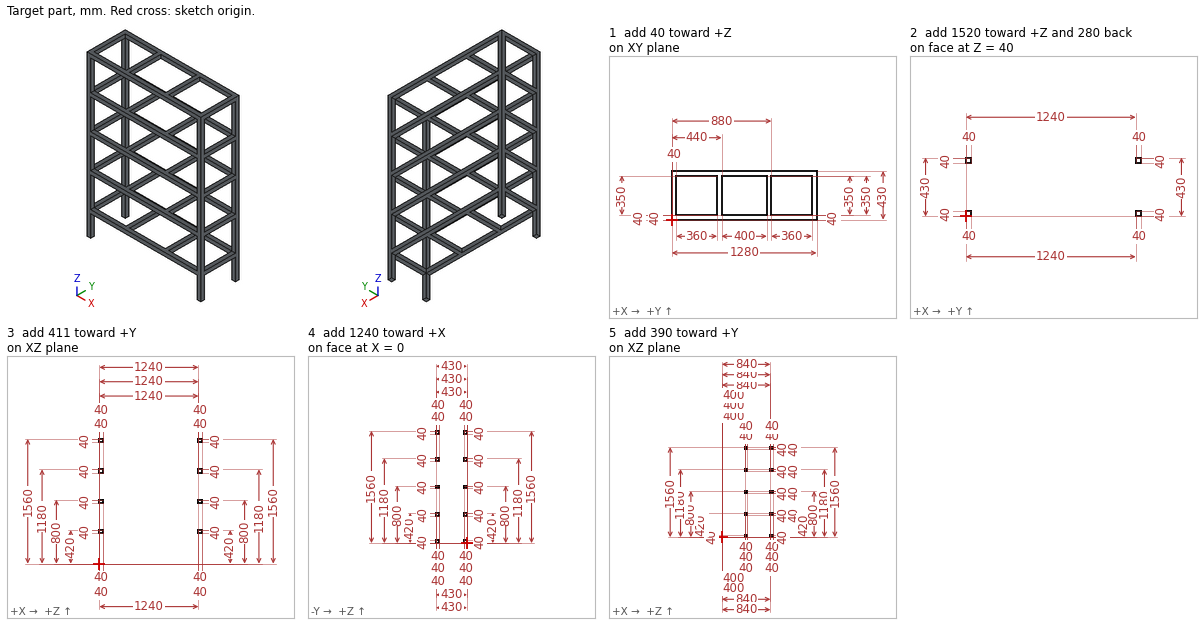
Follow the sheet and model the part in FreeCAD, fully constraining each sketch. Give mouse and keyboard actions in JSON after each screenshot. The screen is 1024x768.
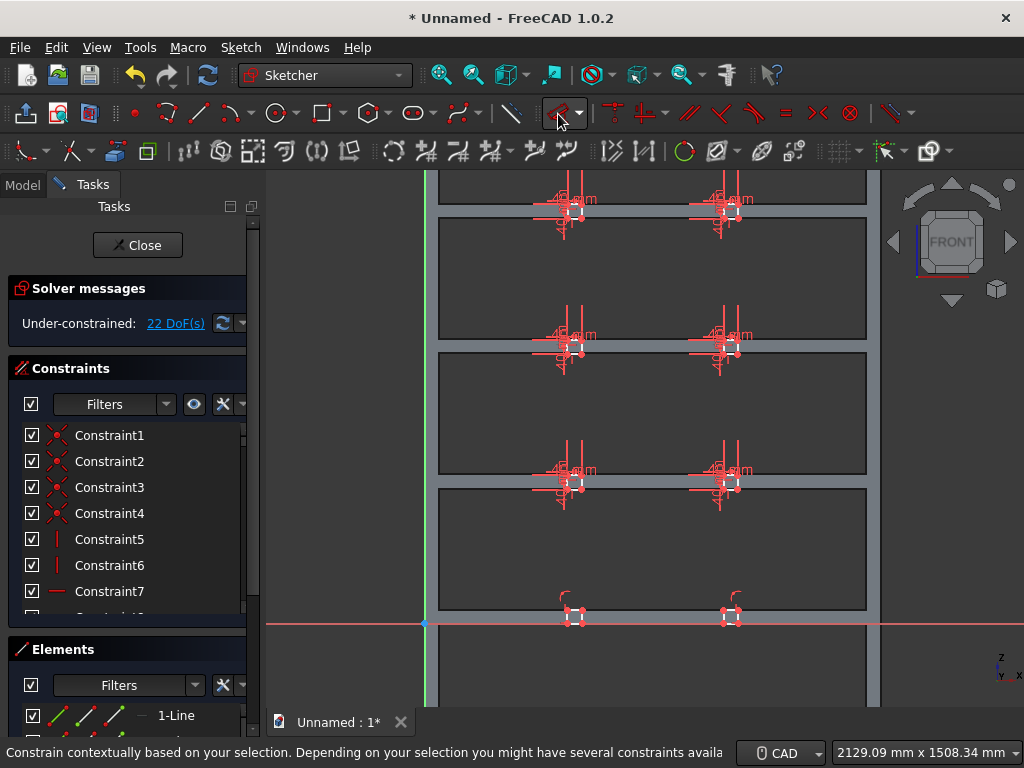
{"action": "scroll", "coordinate": [567, 617], "scroll_direction": "up", "scroll_amount": 6}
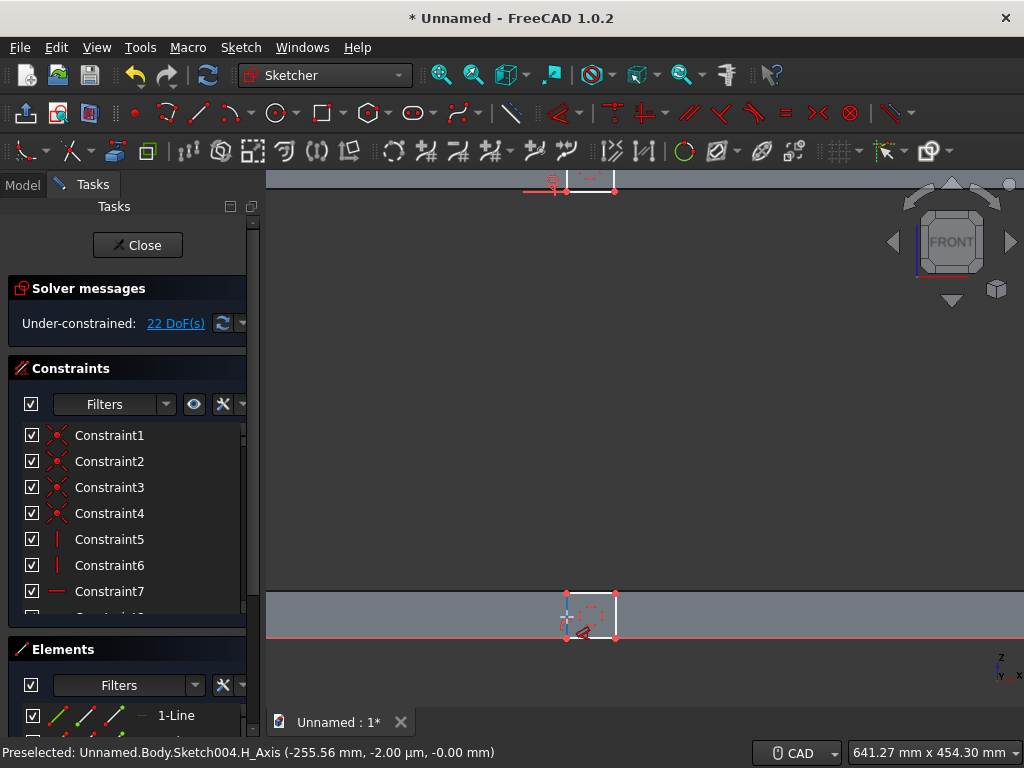
{"action": "left_click", "coordinate": [567, 616]}
{"action": "left_click", "coordinate": [533, 616]}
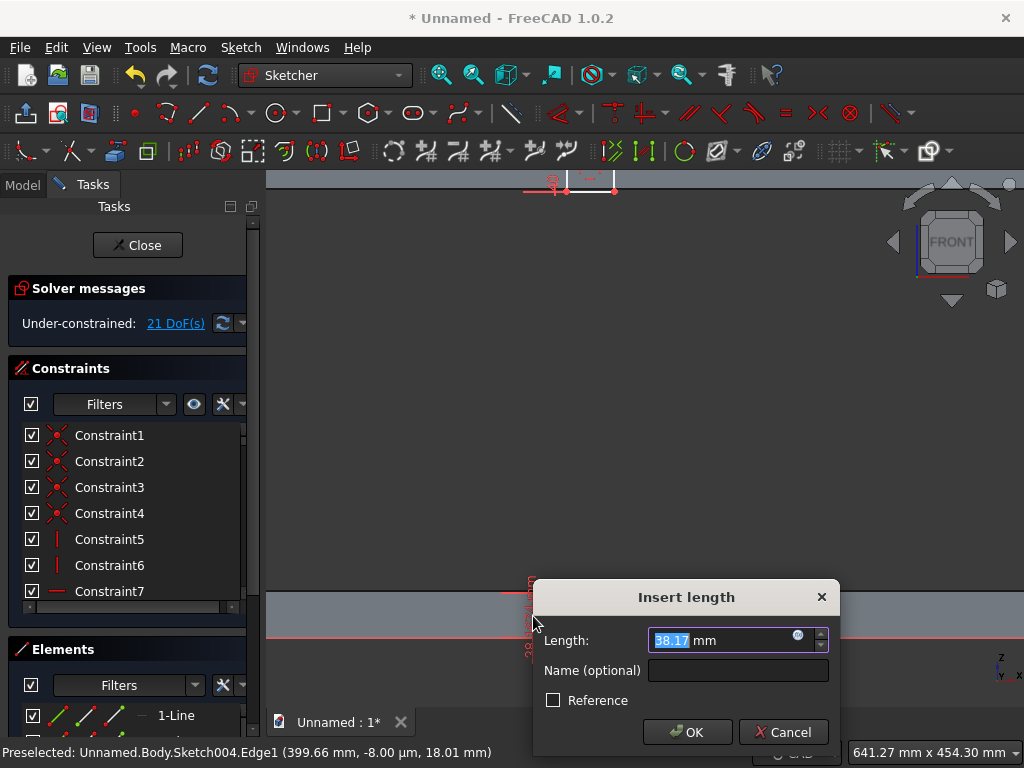
{"action": "type", "text": "40"}
{"action": "key", "text": "Return"}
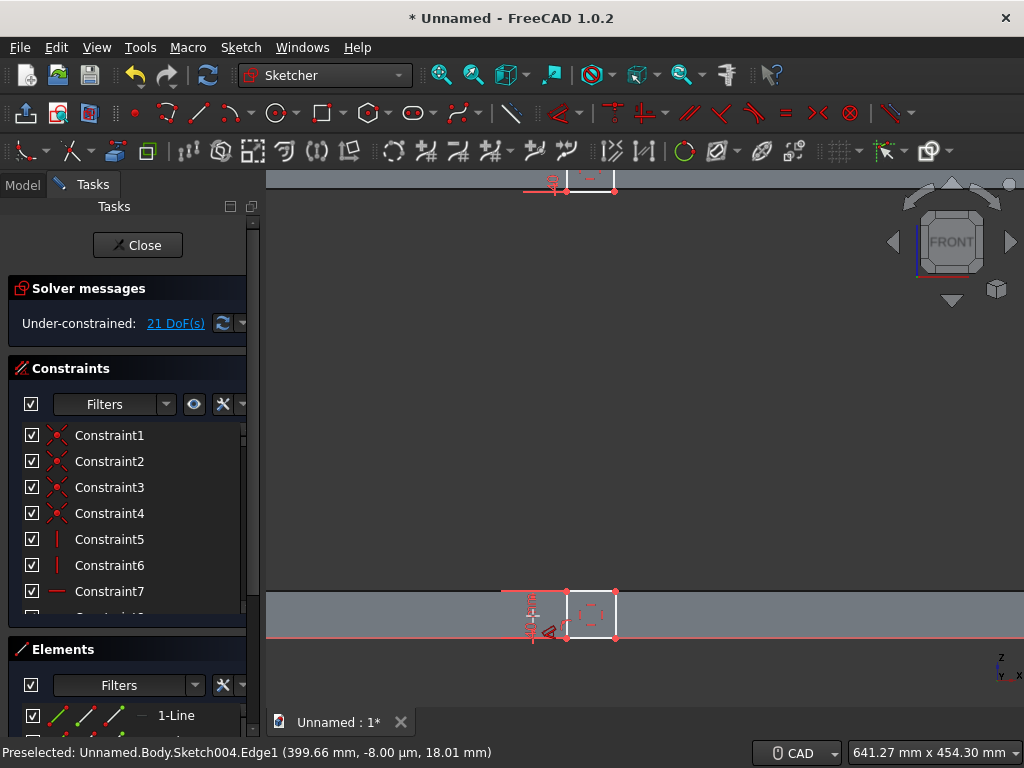
{"action": "left_click", "coordinate": [582, 638]}
{"action": "left_click", "coordinate": [591, 672]}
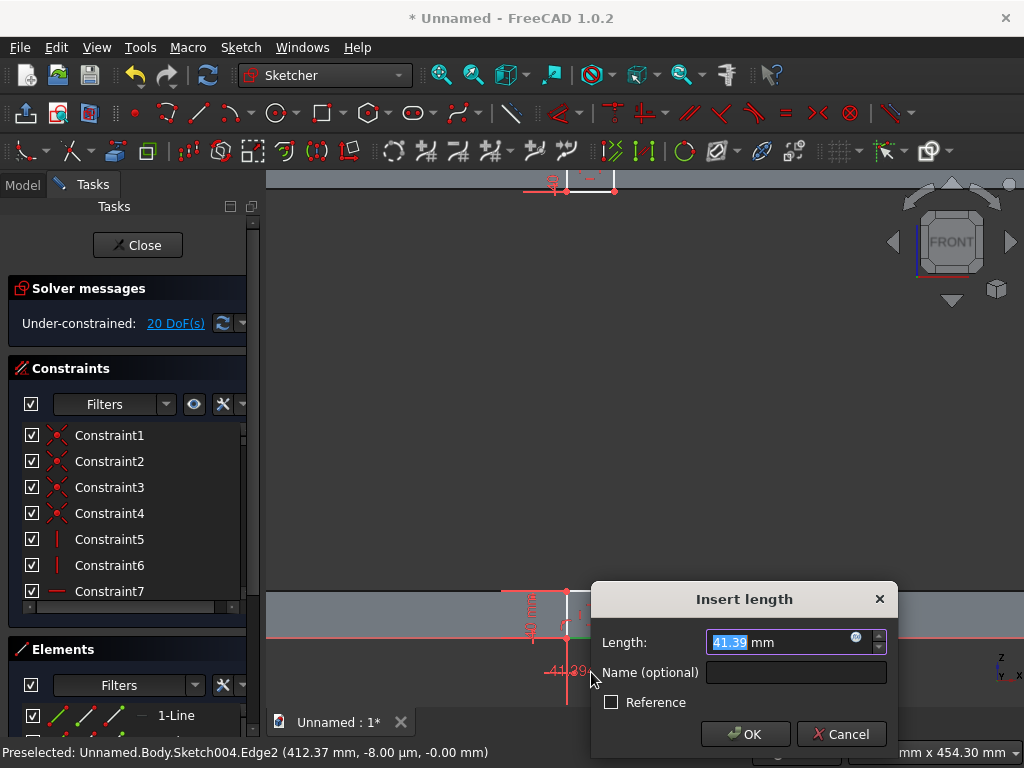
{"action": "type", "text": "40"}
{"action": "key", "text": "Return"}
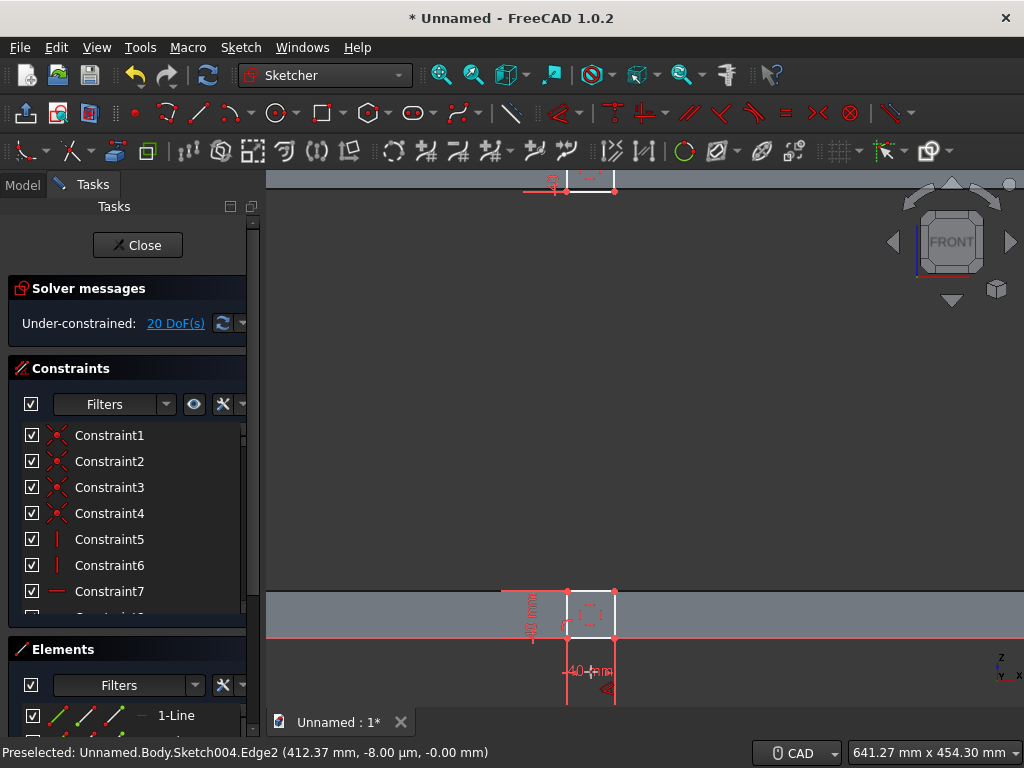
{"action": "scroll", "coordinate": [567, 621], "scroll_direction": "down", "scroll_amount": 8}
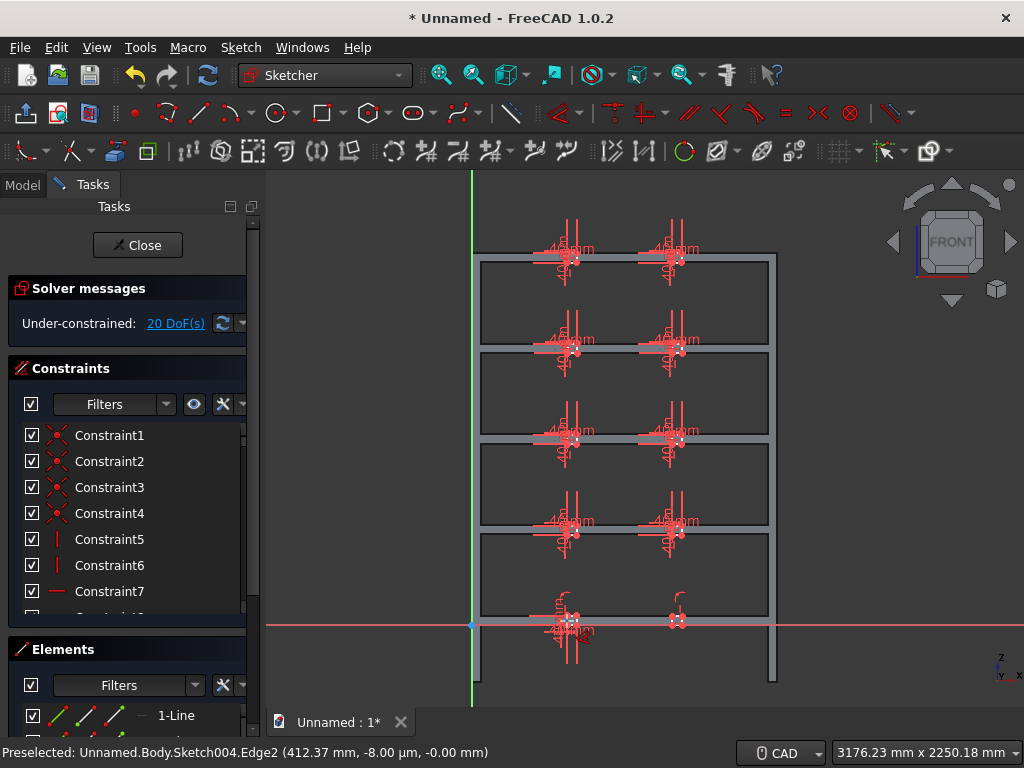
{"action": "scroll", "coordinate": [672, 619], "scroll_direction": "up", "scroll_amount": 9}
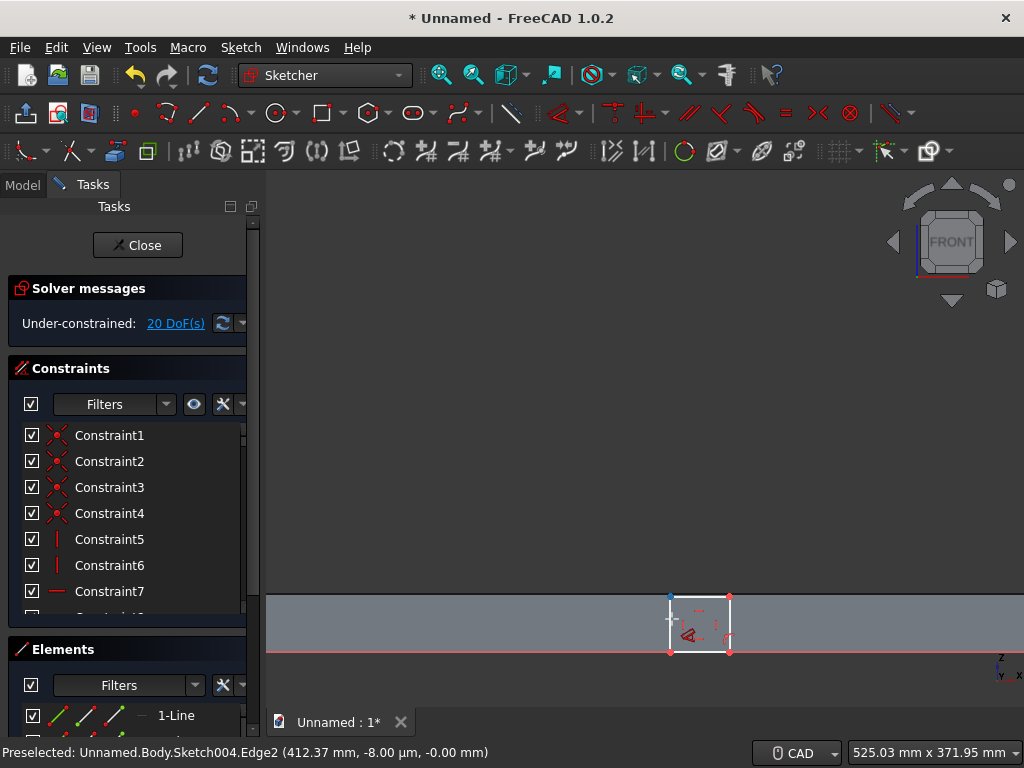
{"action": "left_click", "coordinate": [670, 613]}
{"action": "left_click", "coordinate": [704, 625]}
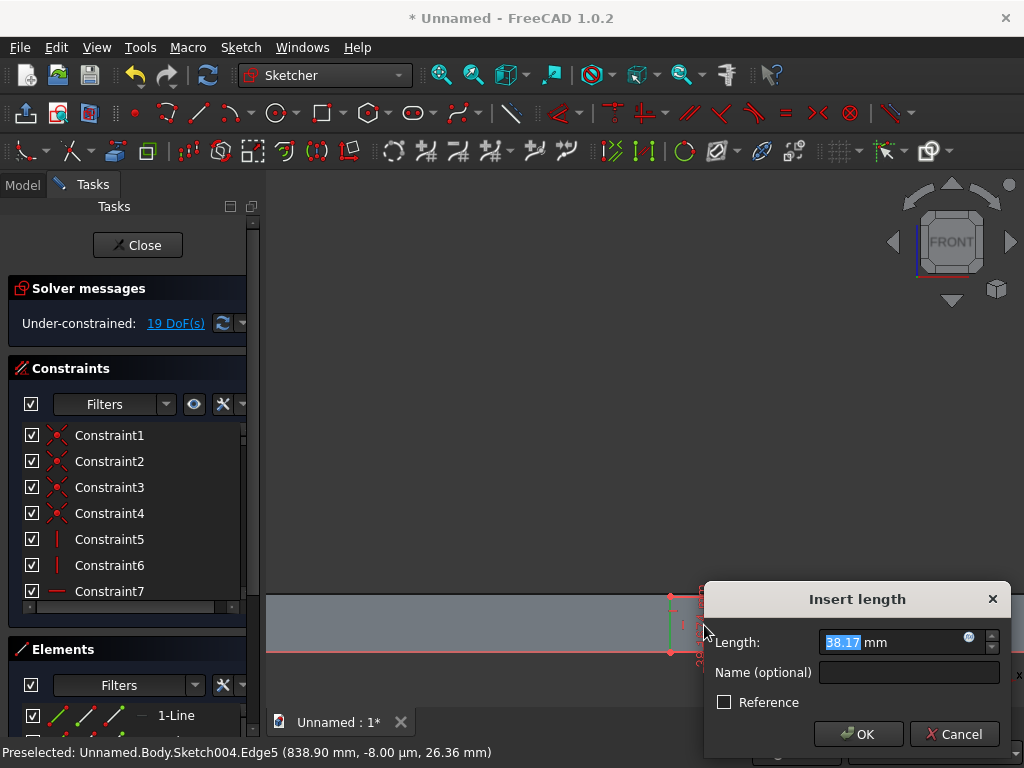
{"action": "type", "text": "40"}
{"action": "key", "text": "Return"}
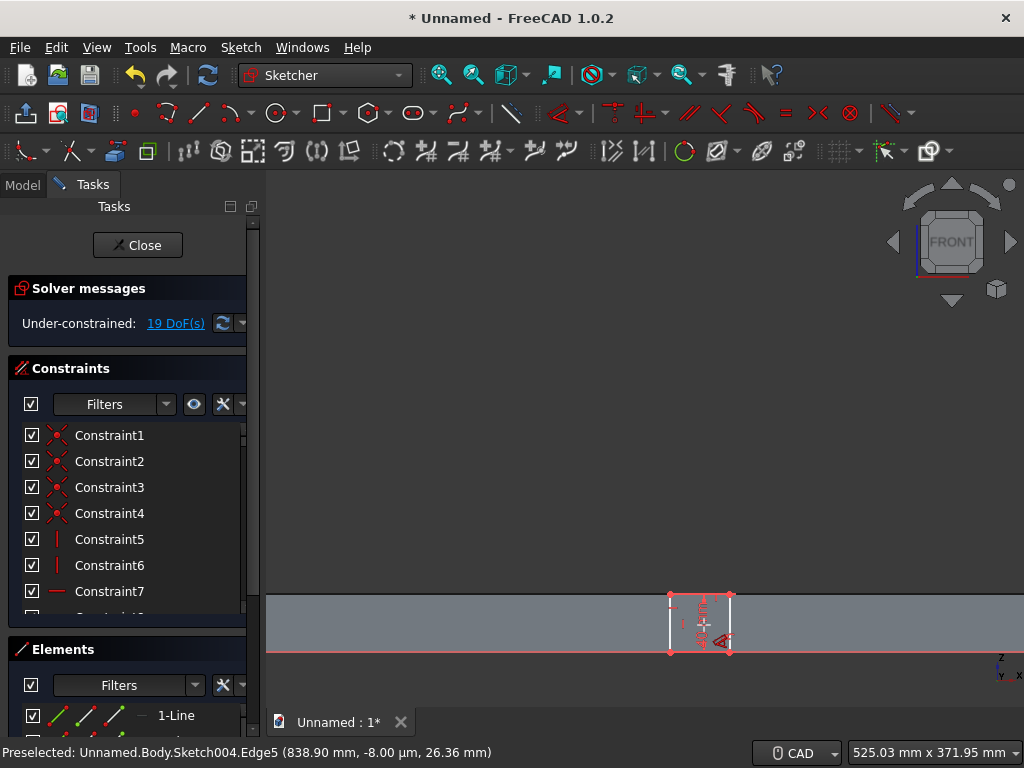
{"action": "left_click", "coordinate": [688, 652]}
{"action": "left_click", "coordinate": [700, 570]}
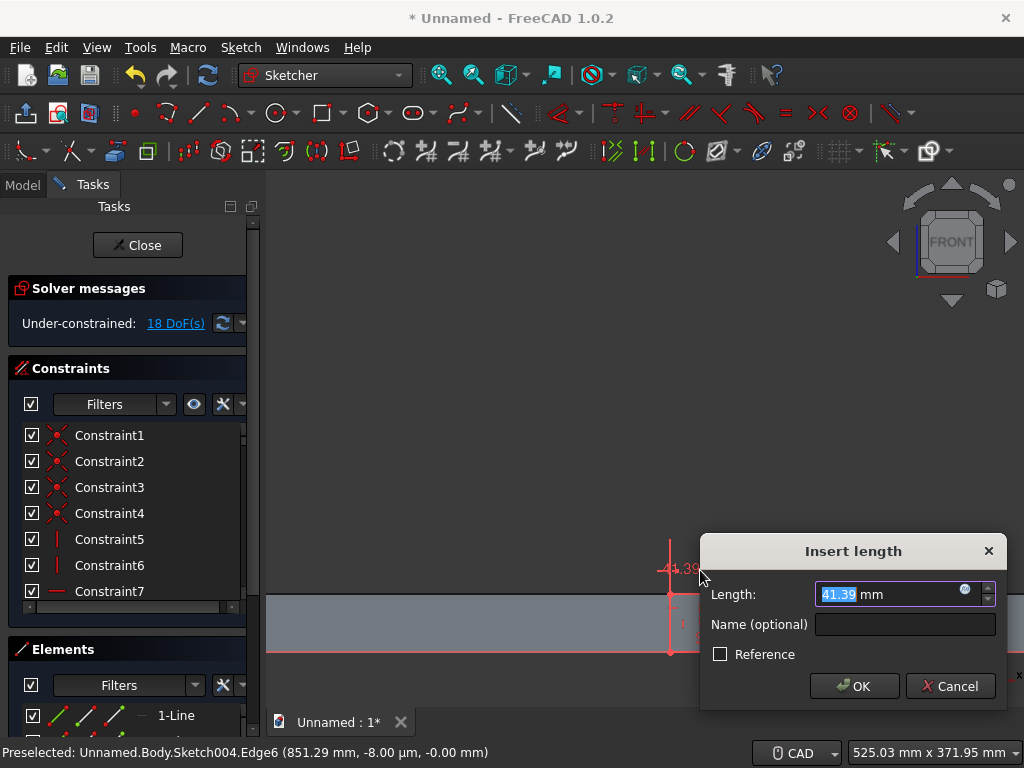
{"action": "type", "text": "40"}
{"action": "key", "text": "Return"}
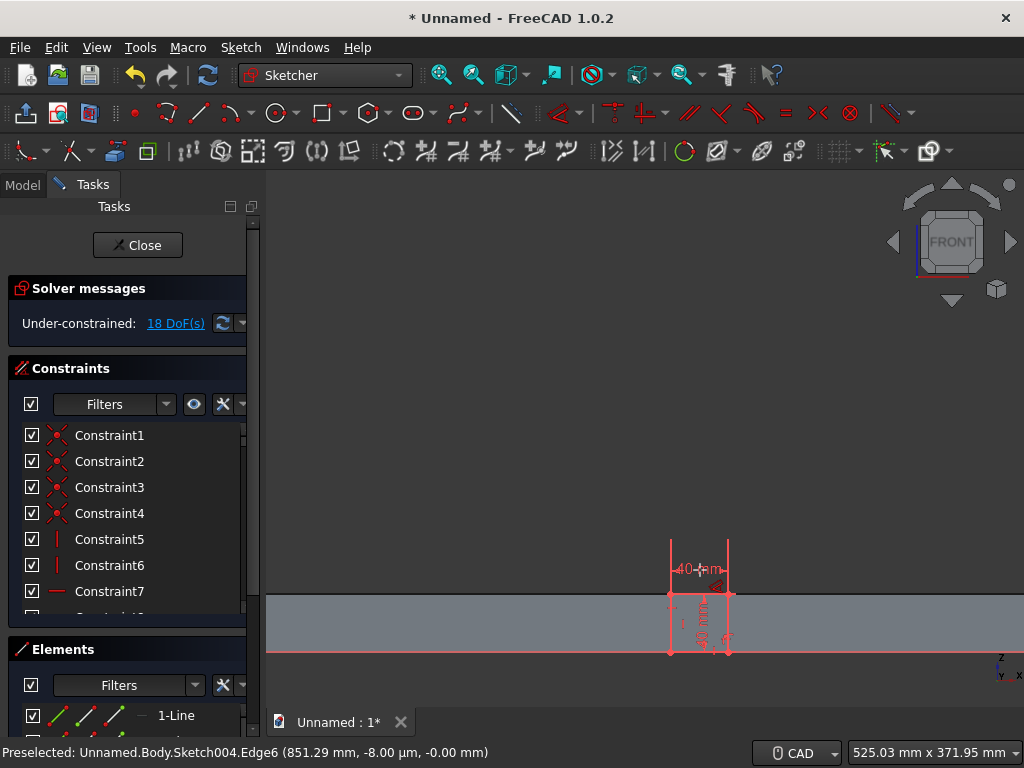
{"action": "scroll", "coordinate": [672, 619], "scroll_direction": "down", "scroll_amount": 9}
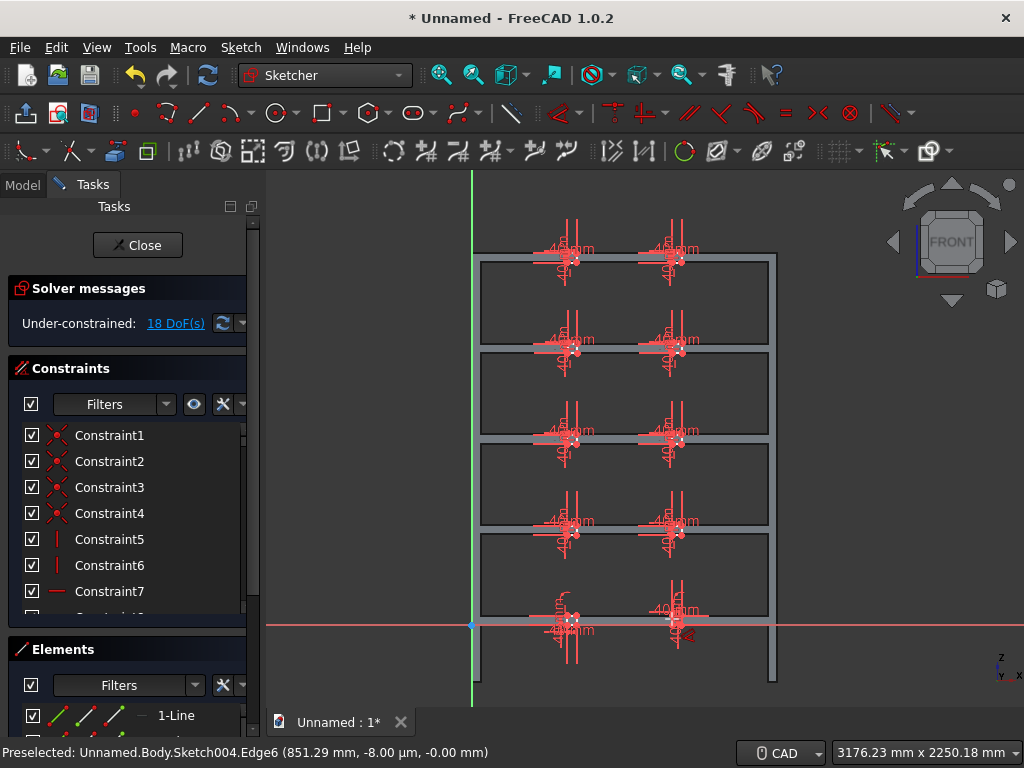
{"action": "scroll", "coordinate": [567, 616], "scroll_direction": "up", "scroll_amount": 2}